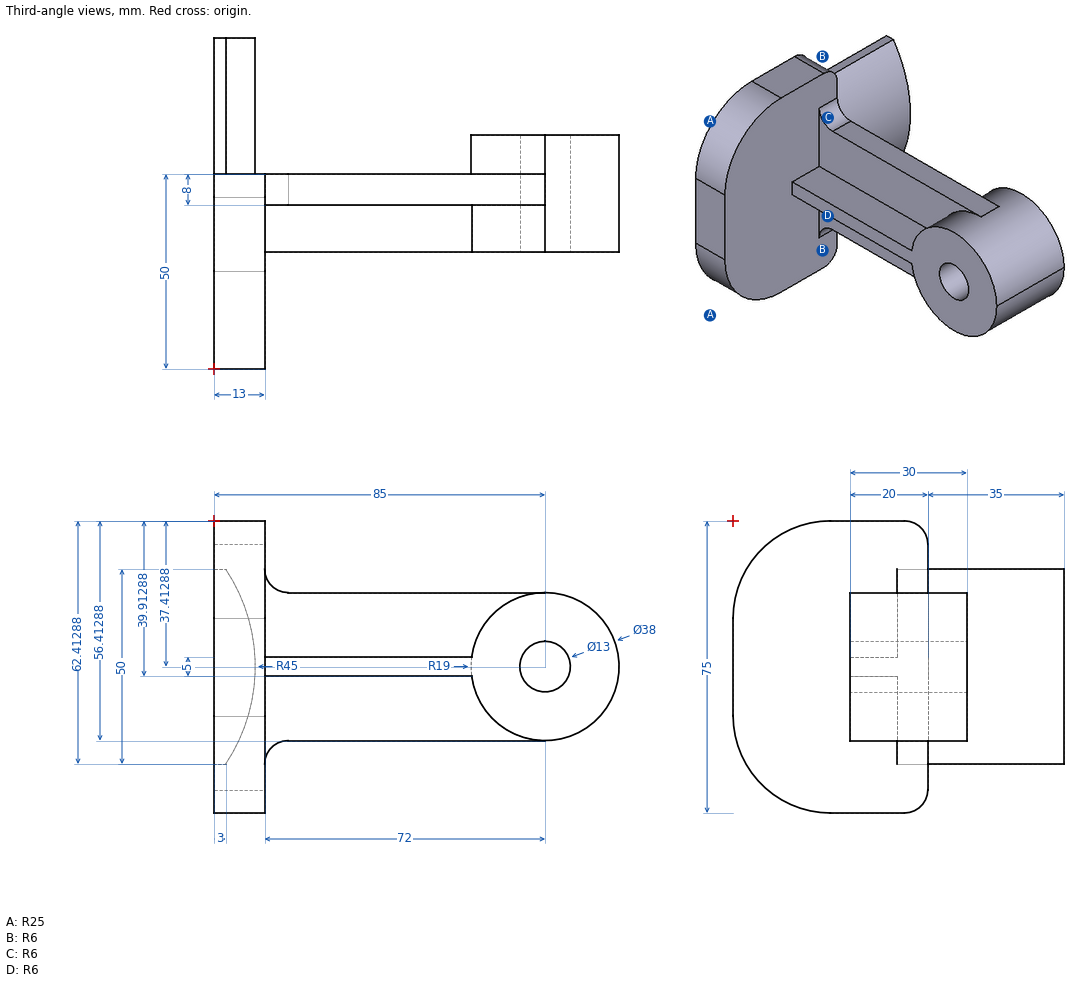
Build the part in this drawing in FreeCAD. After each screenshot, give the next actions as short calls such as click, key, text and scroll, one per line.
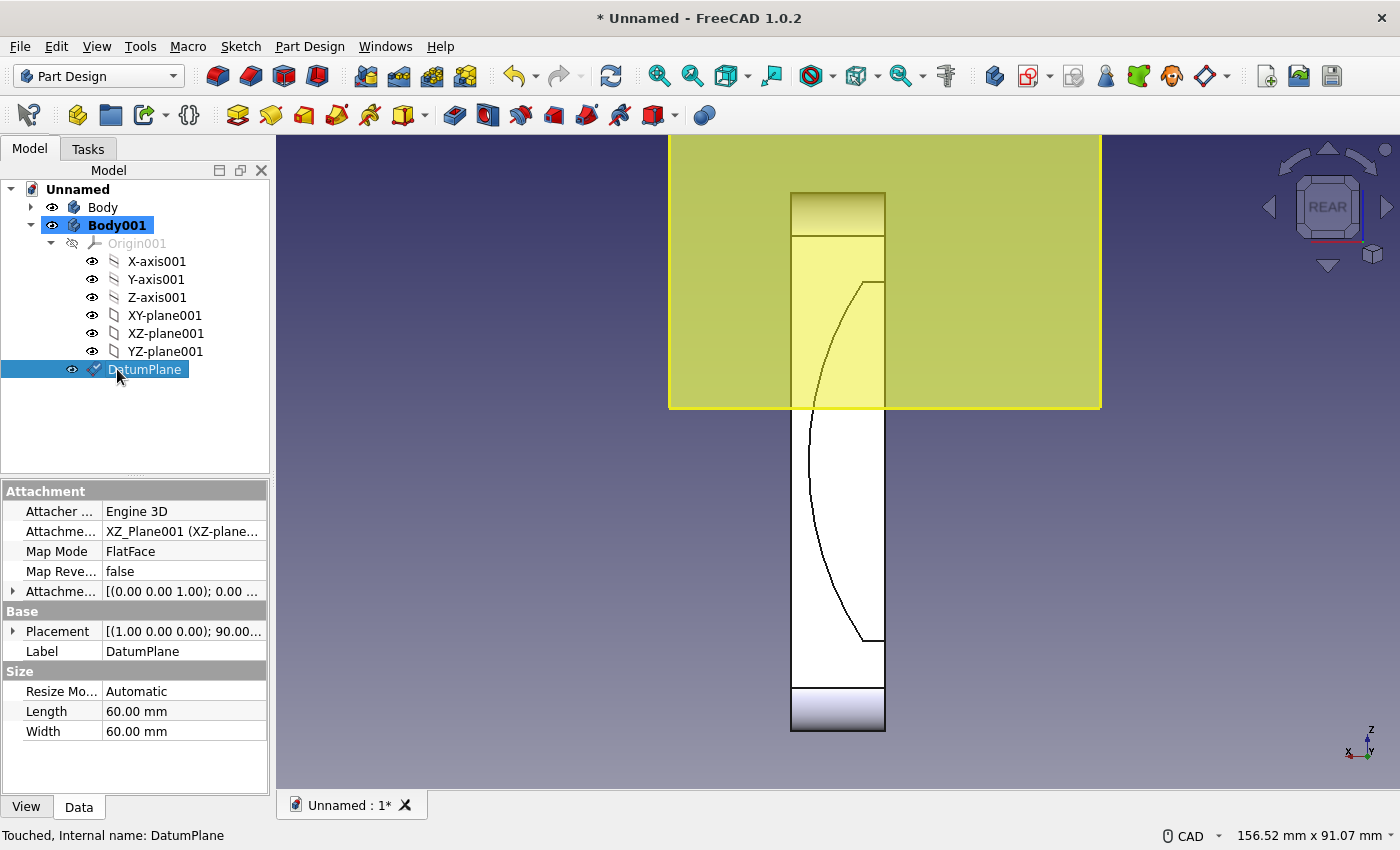
click(1028, 76)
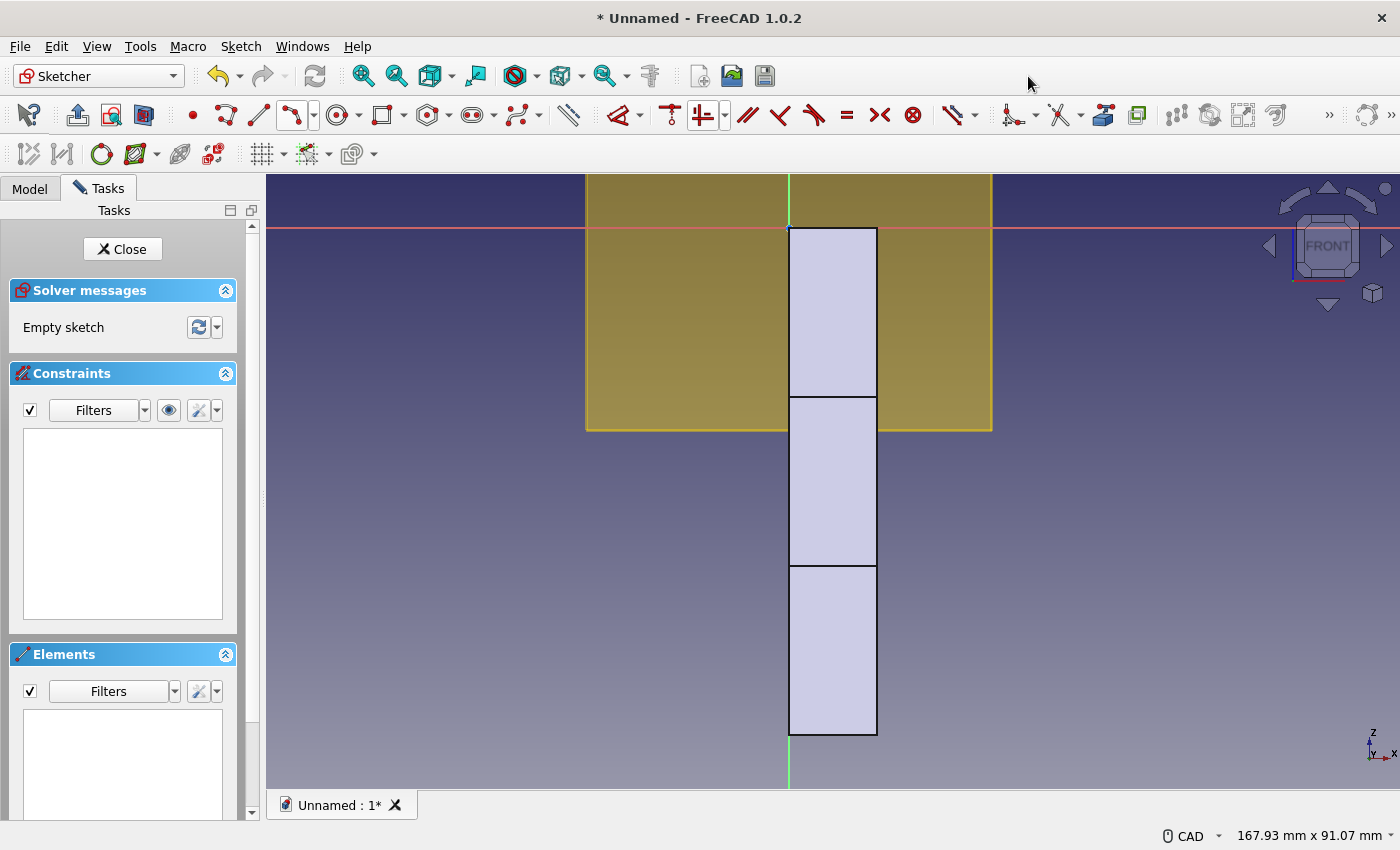
scroll(764, 482, down, 5)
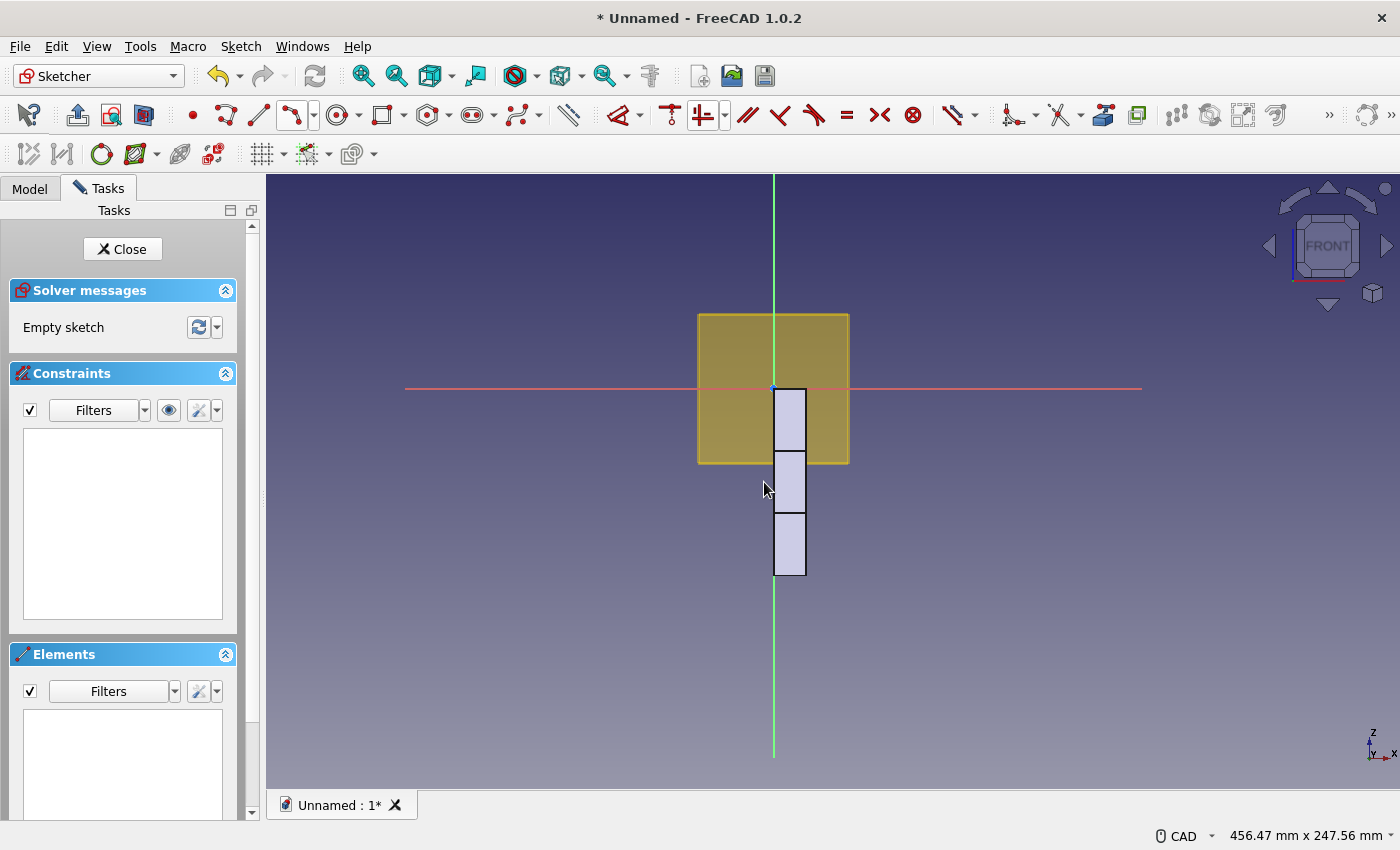
scroll(1057, 482, up, 7)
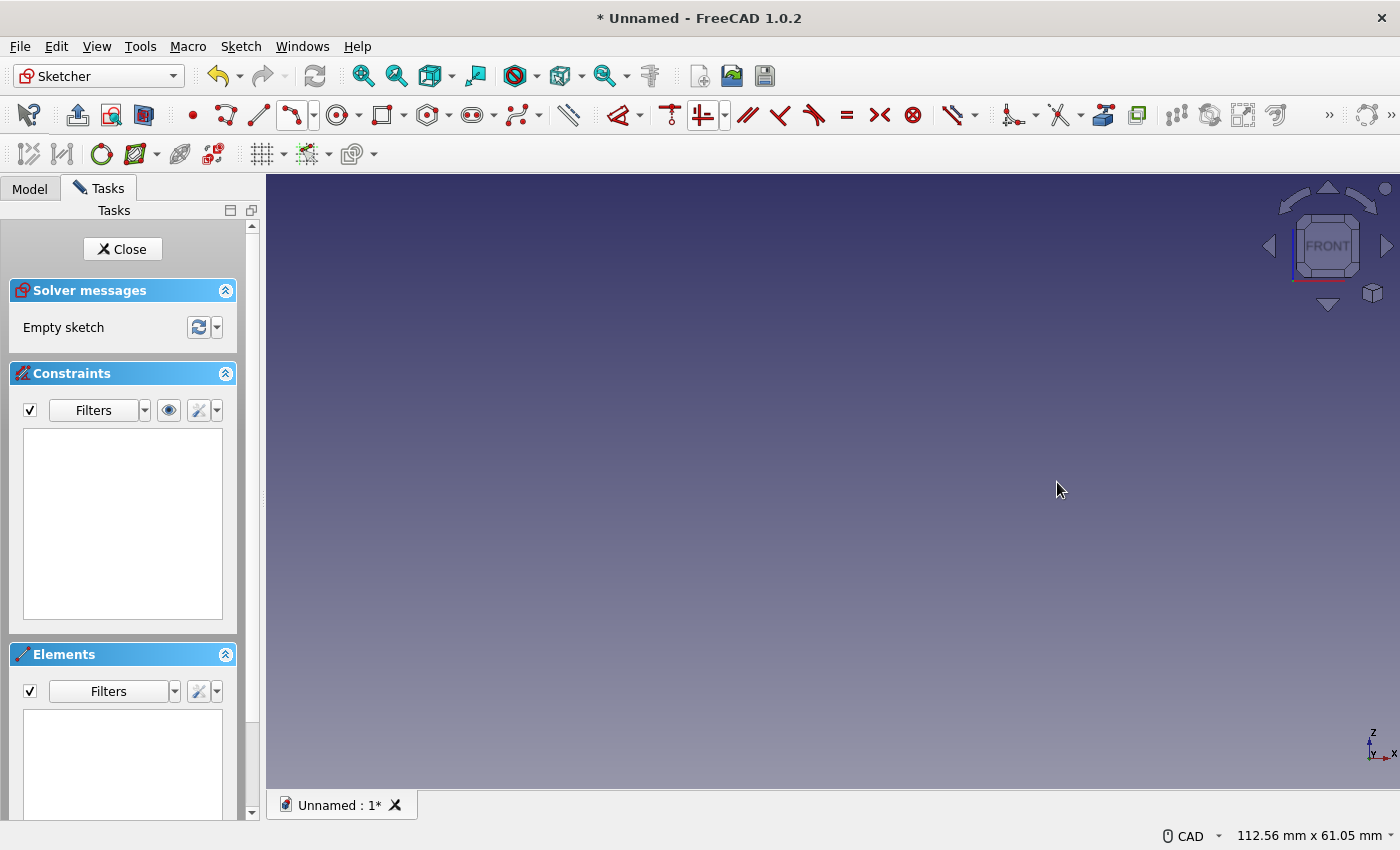
click(336, 116)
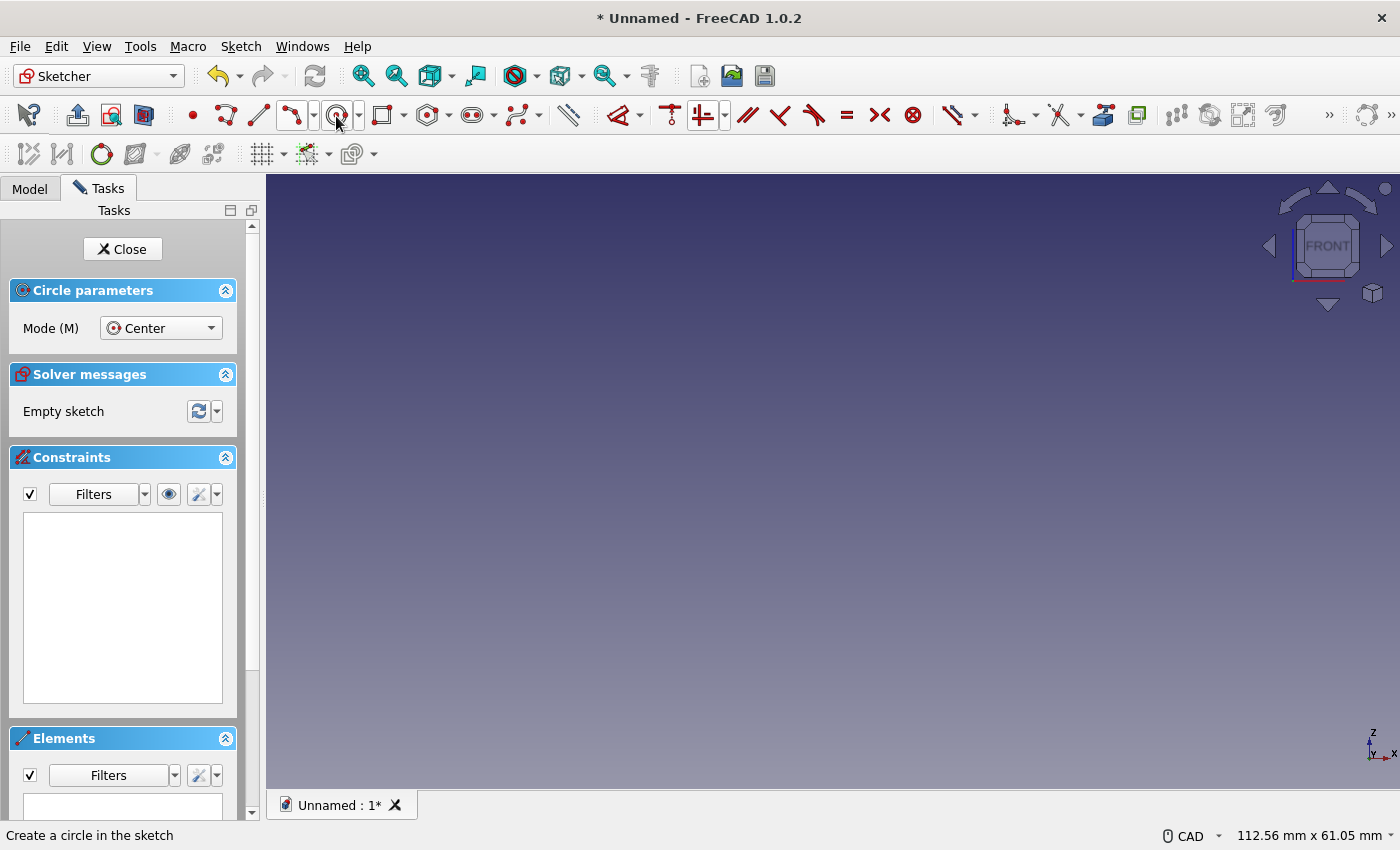
click(762, 480)
click(897, 345)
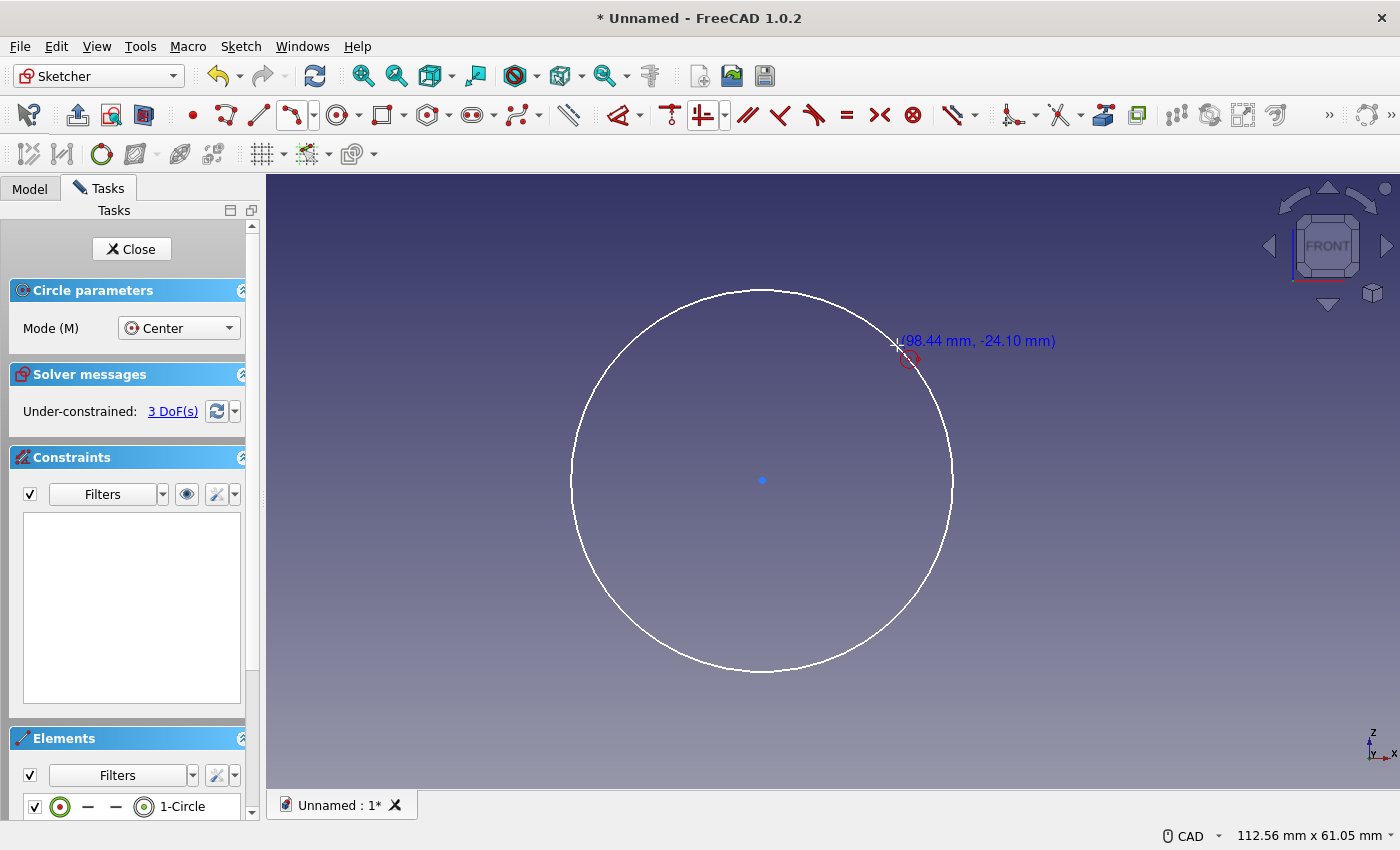
click(762, 481)
click(808, 434)
key(Escape)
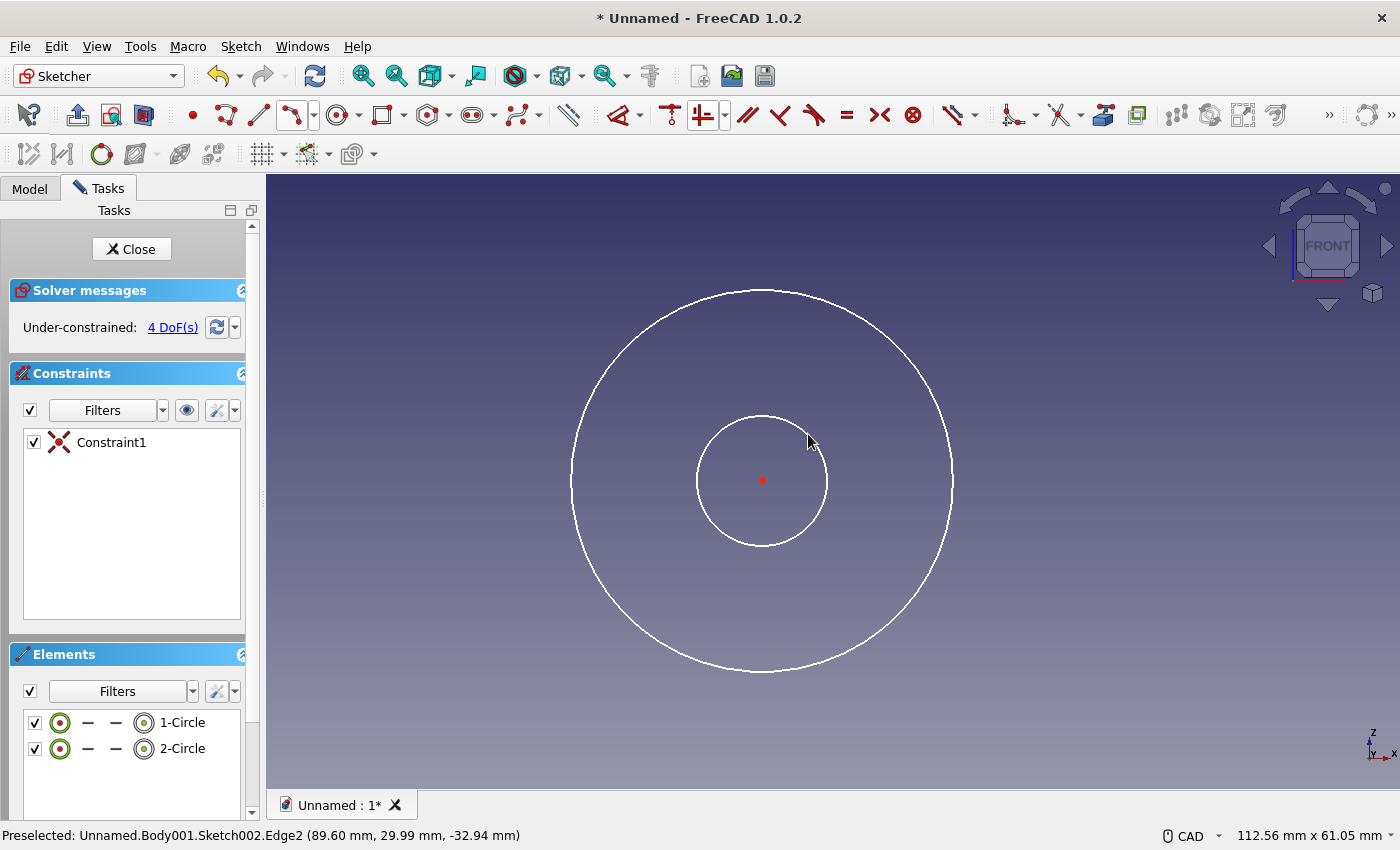
click(618, 116)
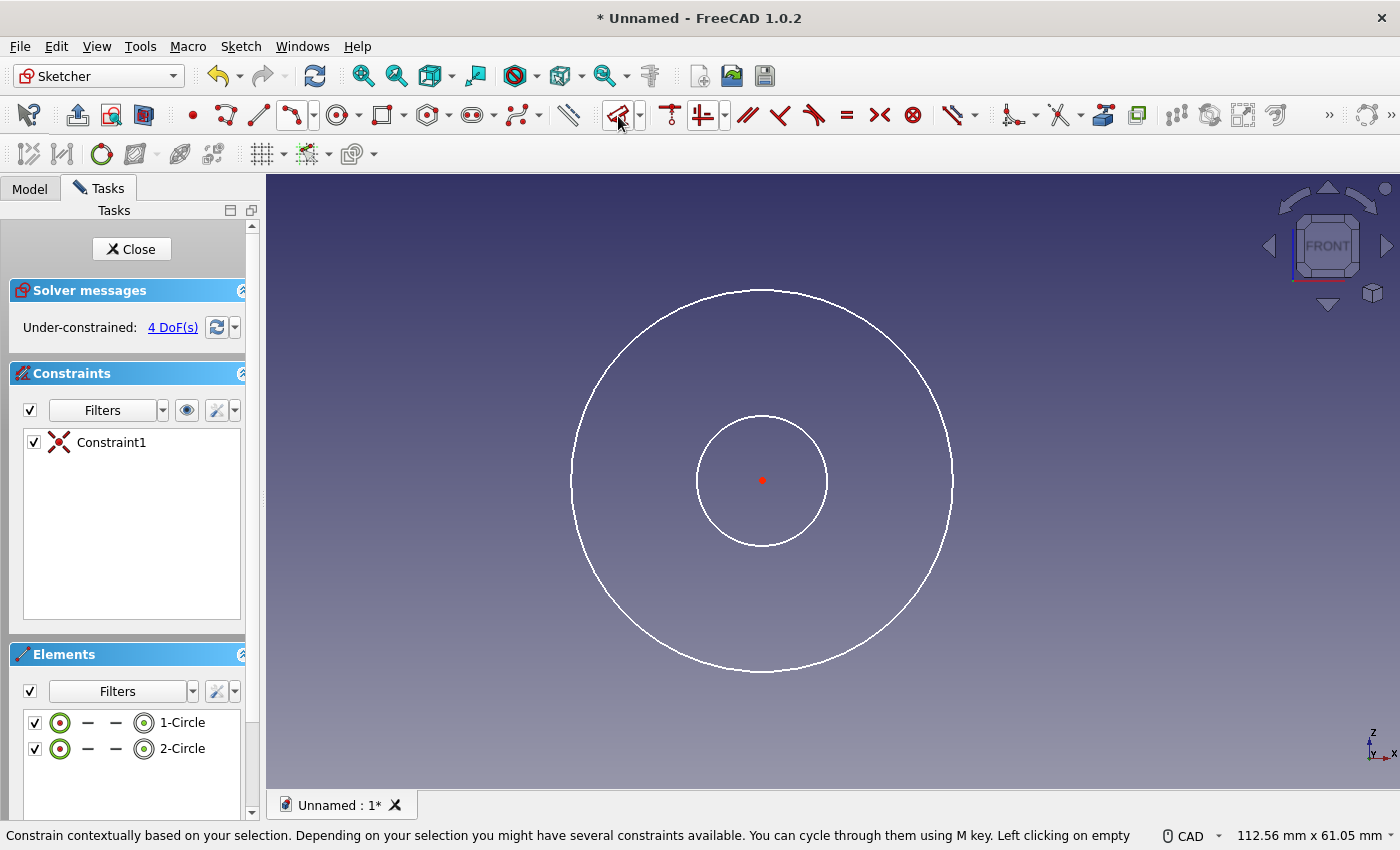
click(897, 346)
click(920, 323)